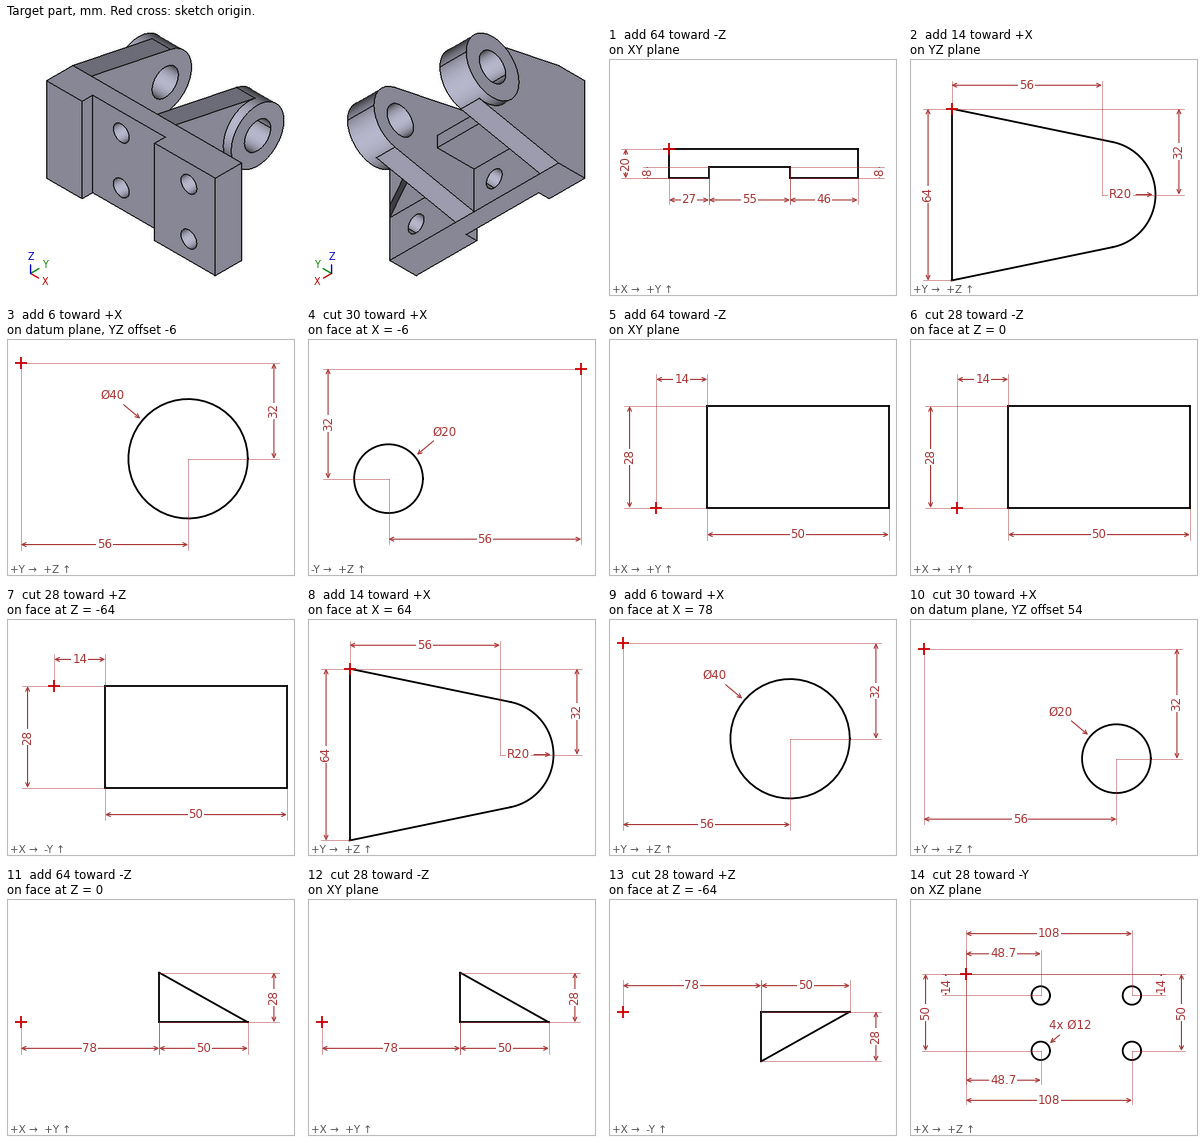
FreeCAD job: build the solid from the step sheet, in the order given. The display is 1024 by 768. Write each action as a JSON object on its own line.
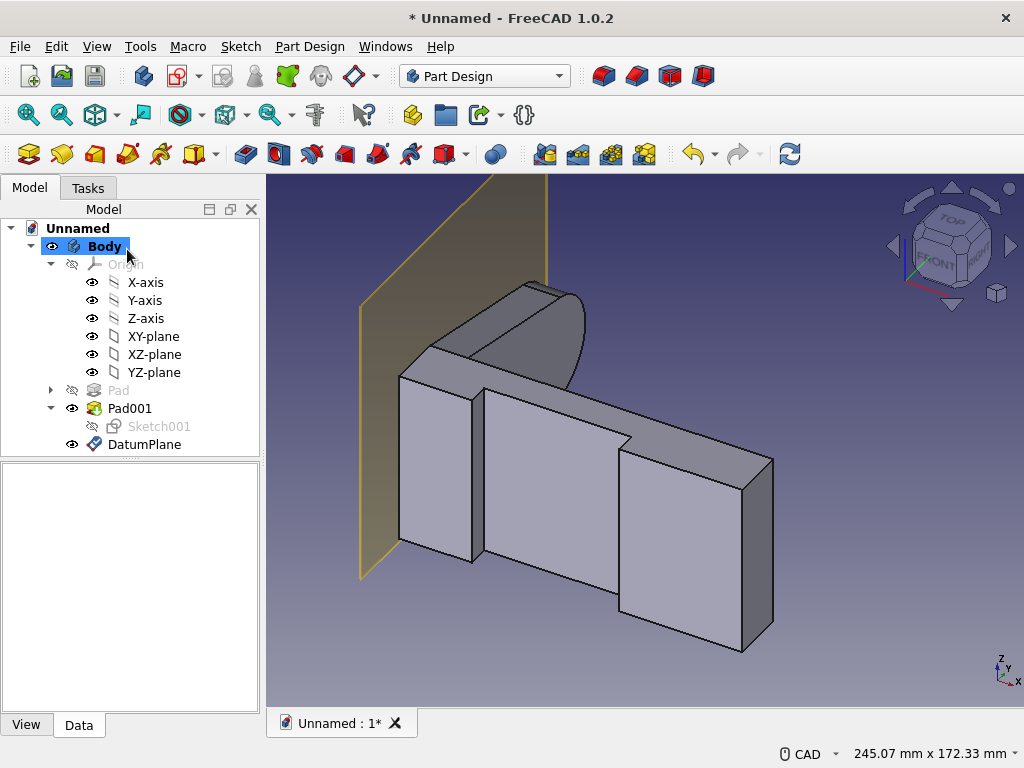
{"action": "left_click", "coordinate": [117, 444]}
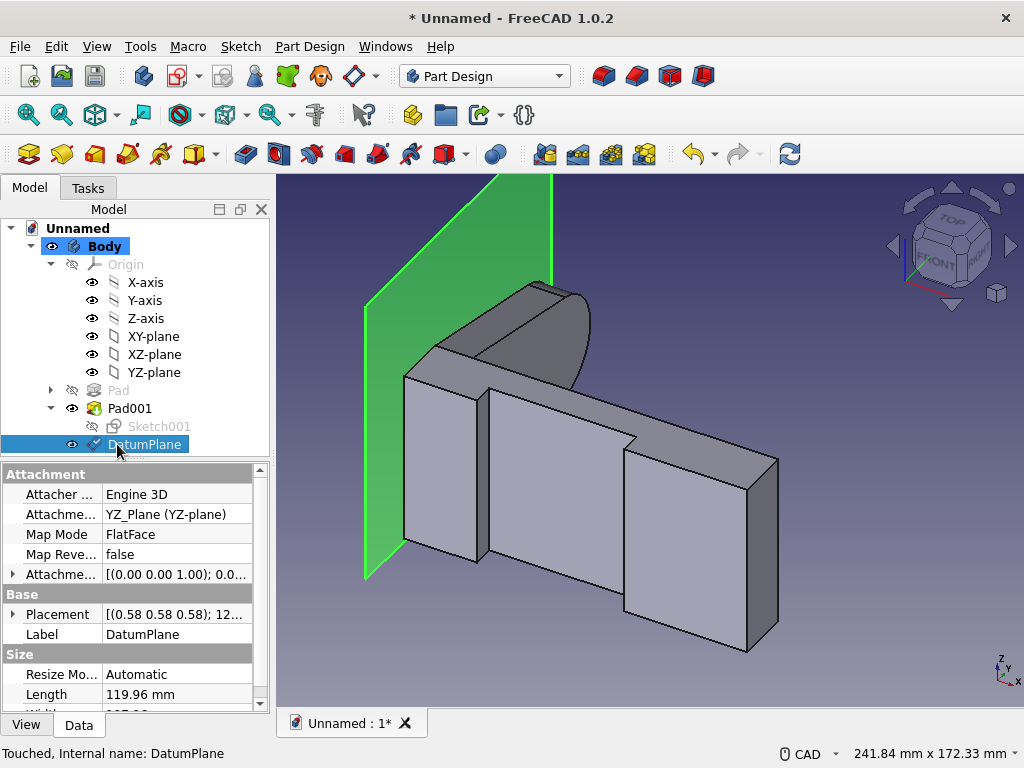
{"action": "left_click", "coordinate": [176, 76]}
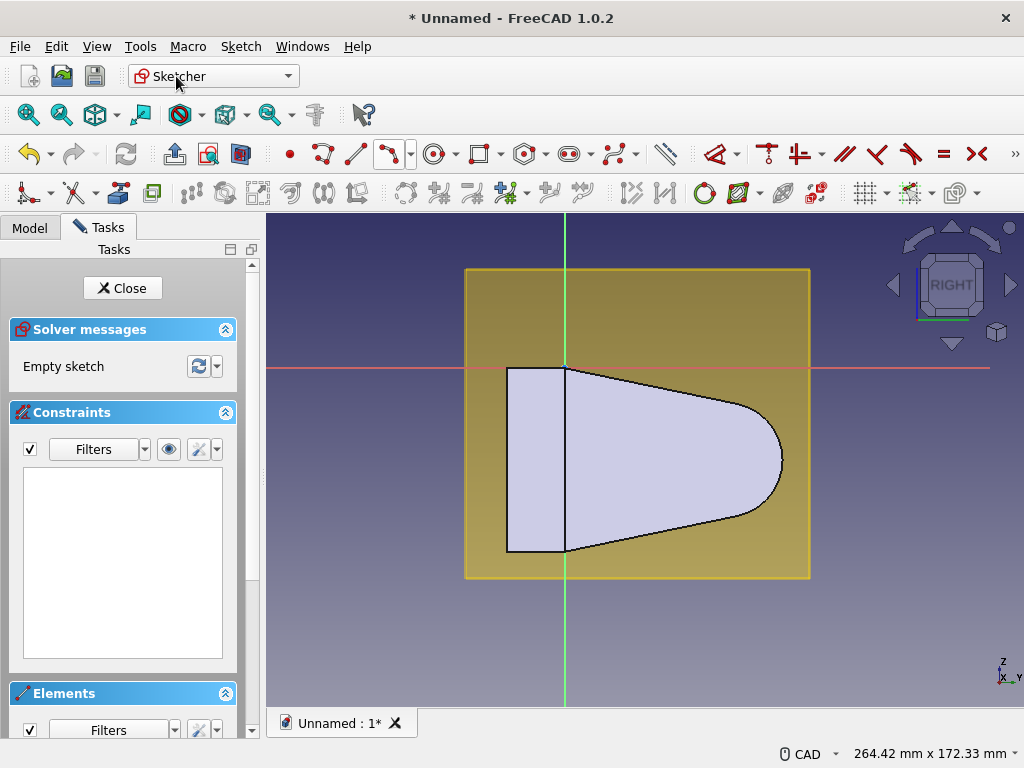
{"action": "left_click", "coordinate": [241, 154]}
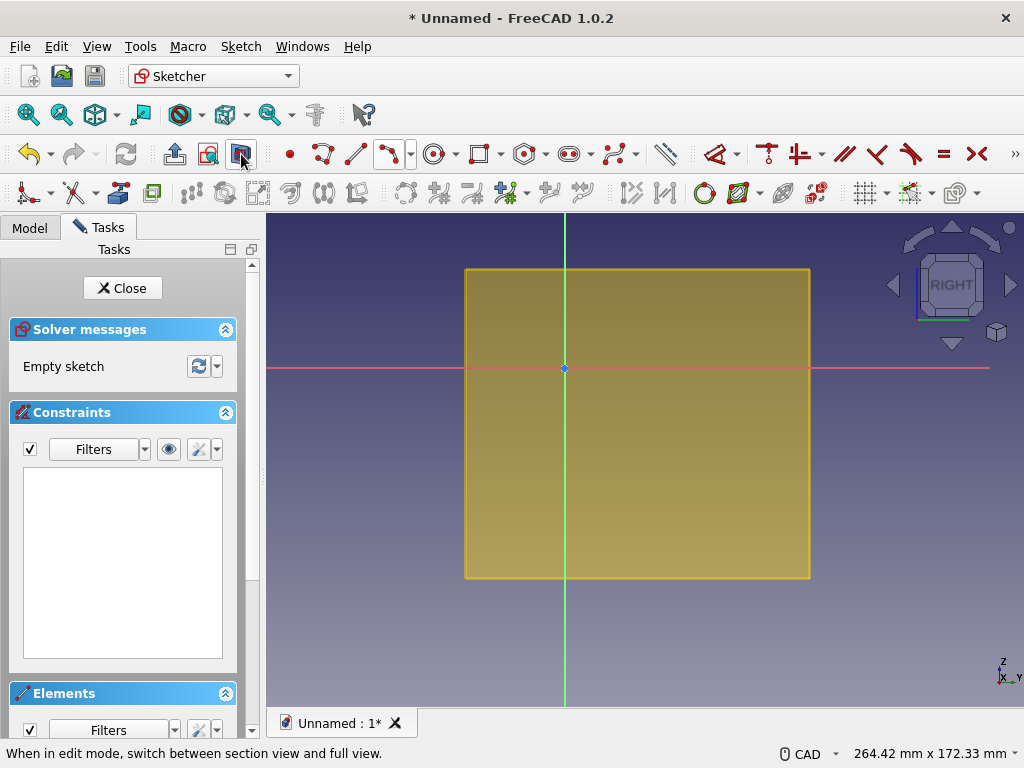
{"action": "scroll", "coordinate": [792, 422], "scroll_direction": "up", "scroll_amount": 3}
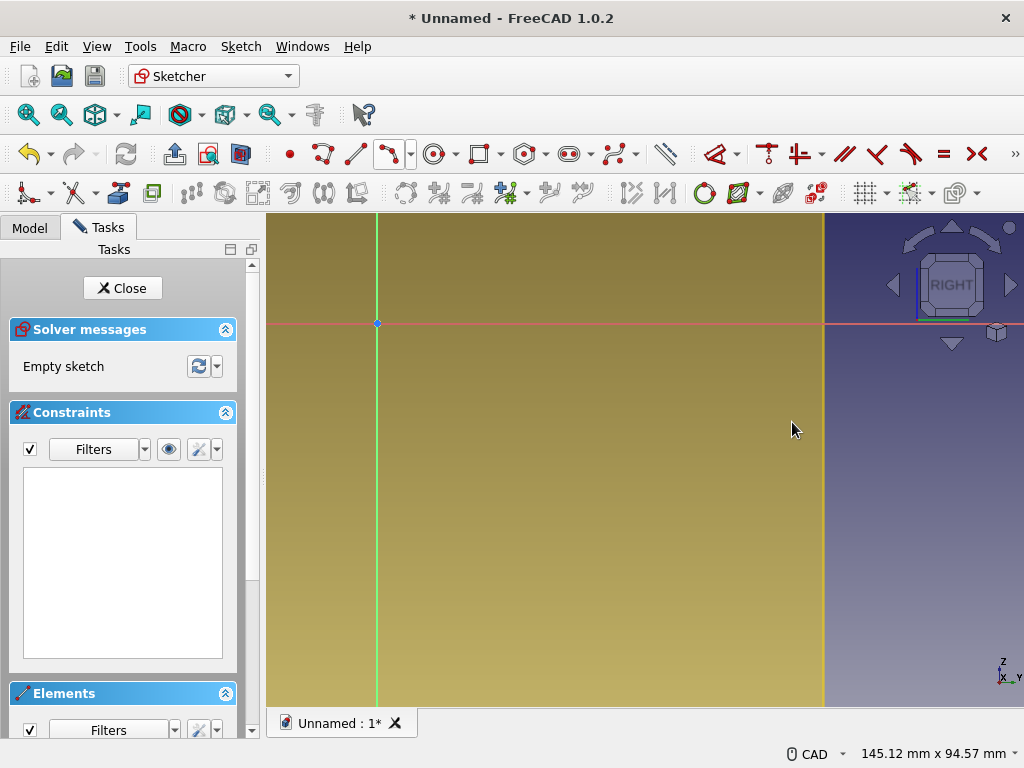
{"action": "left_click", "coordinate": [434, 154]}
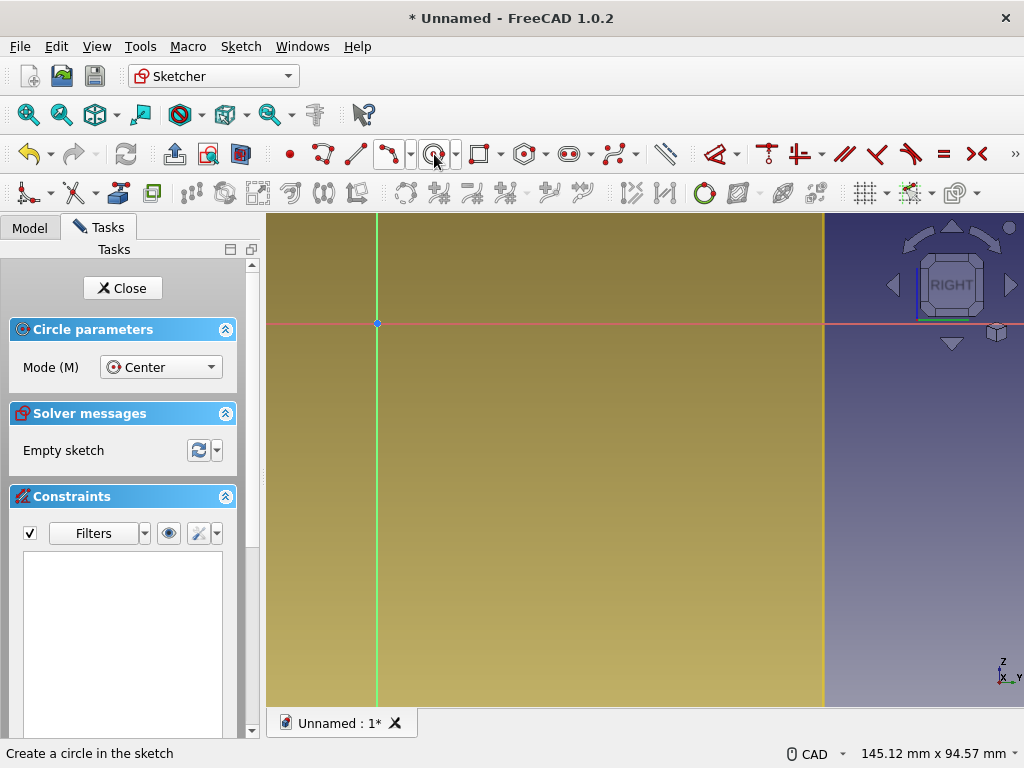
{"action": "left_click", "coordinate": [670, 491]}
{"action": "left_click", "coordinate": [744, 417]}
{"action": "key", "text": "Escape"}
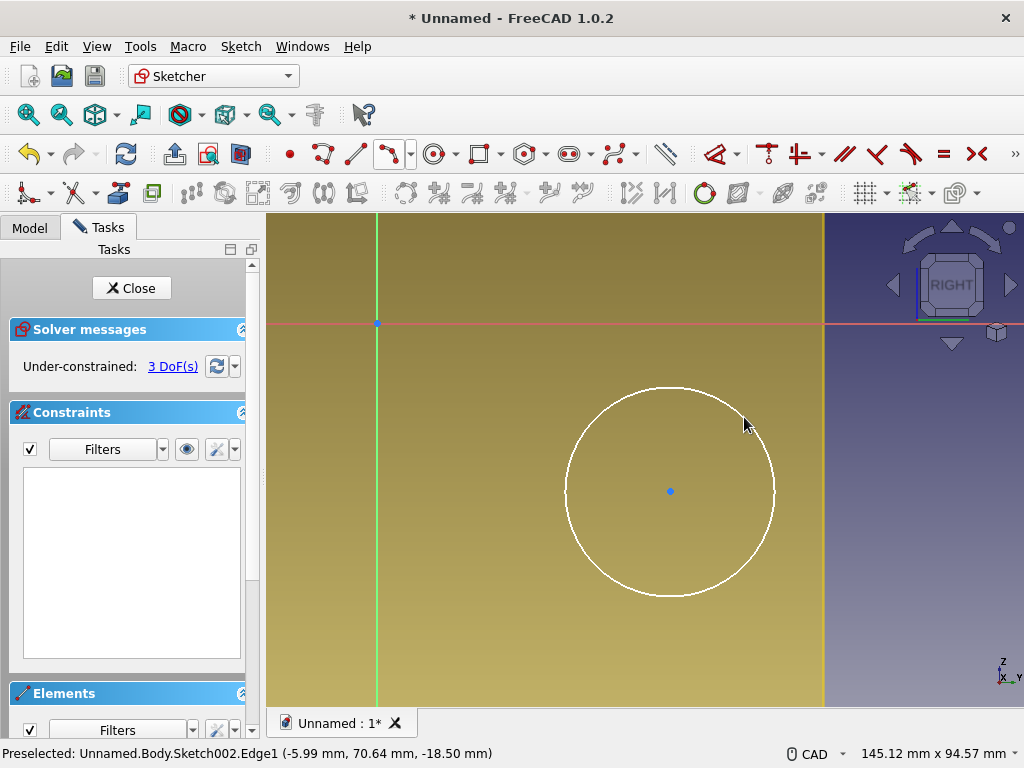
{"action": "left_click", "coordinate": [714, 154]}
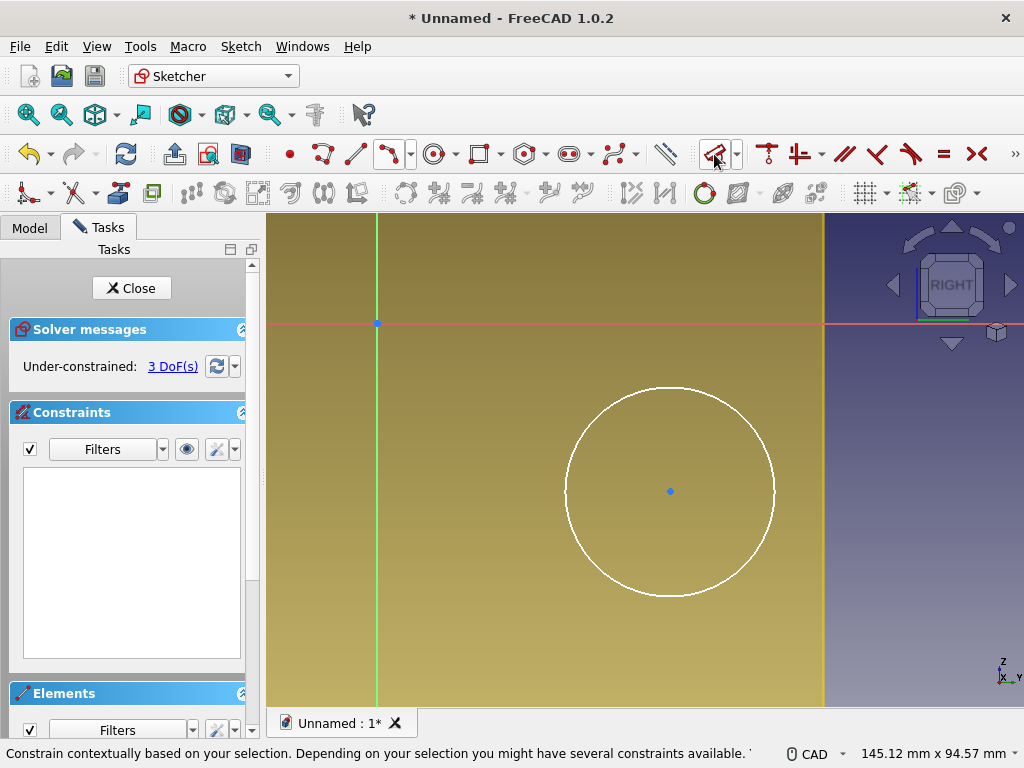
{"action": "left_click", "coordinate": [744, 418]}
{"action": "left_click", "coordinate": [767, 395]}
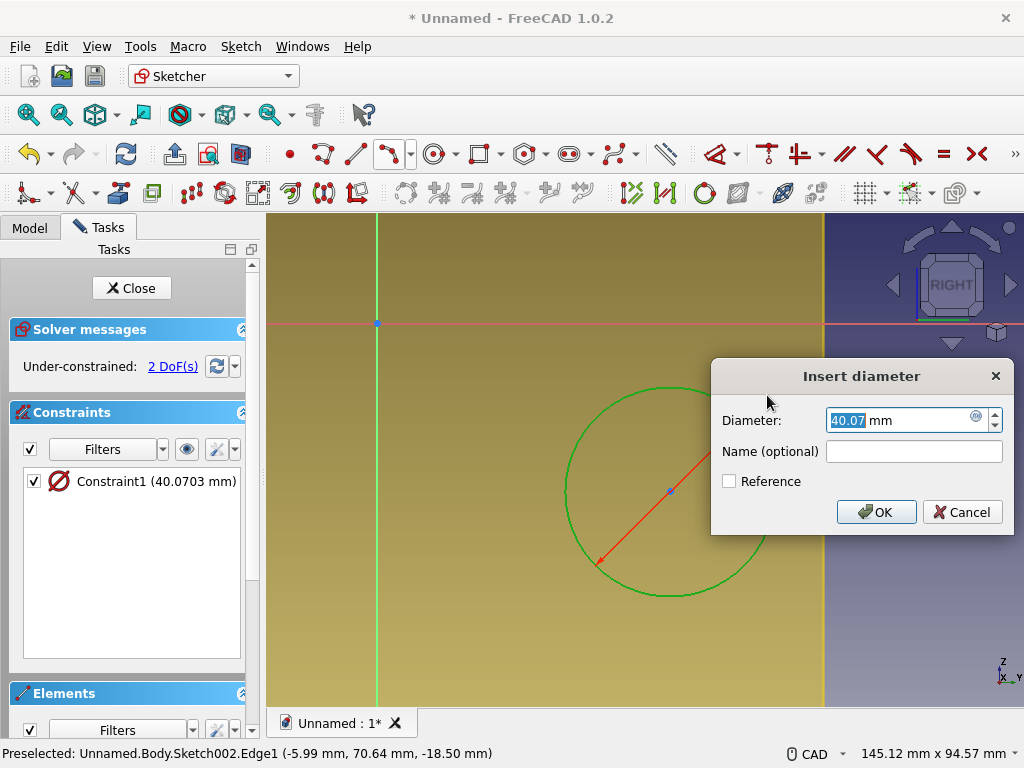
{"action": "type", "text": "40"}
{"action": "key", "text": "Return"}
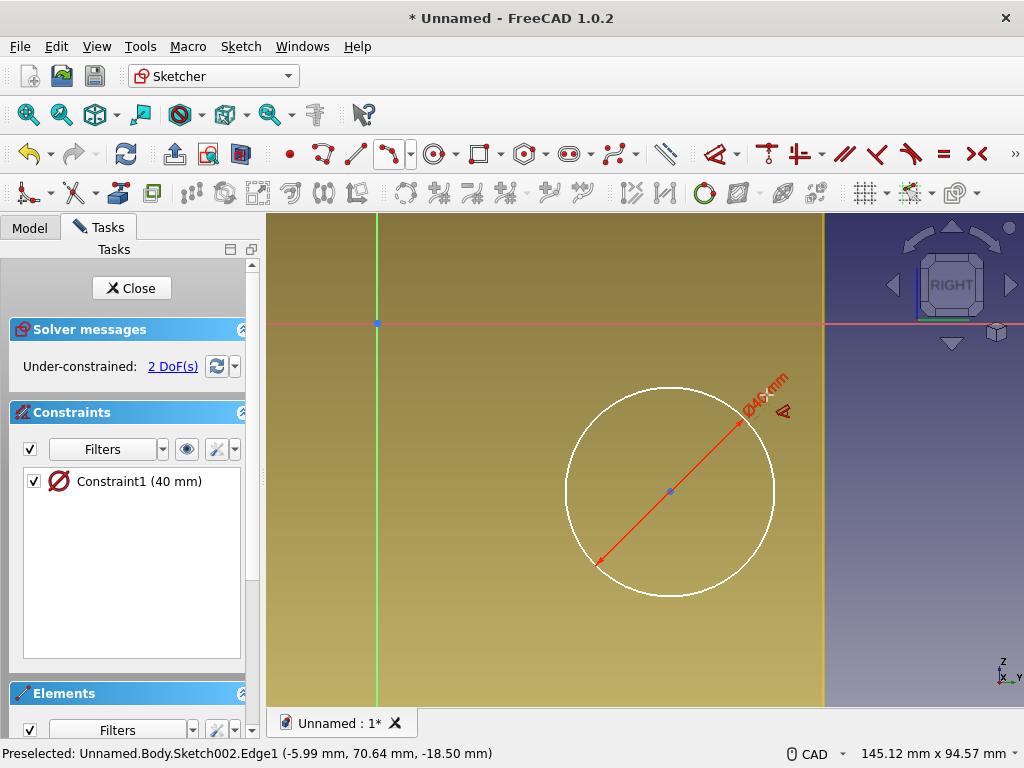
{"action": "left_click", "coordinate": [670, 492]}
{"action": "left_click", "coordinate": [524, 290]}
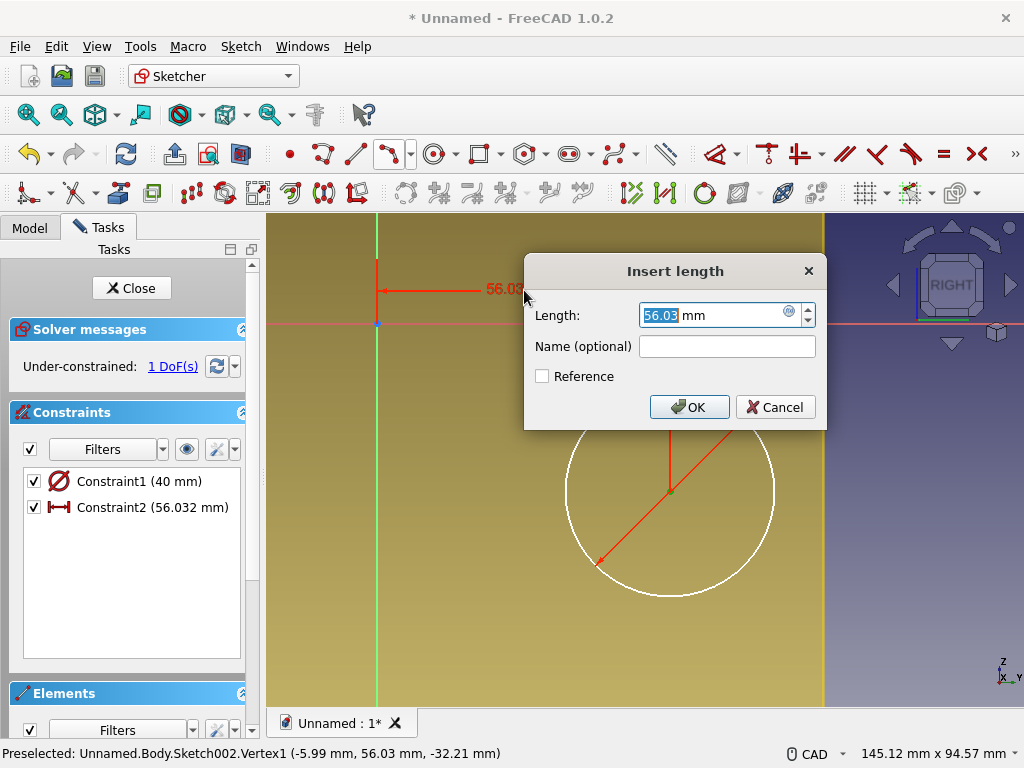
{"action": "type", "text": "56"}
{"action": "key", "text": "Return"}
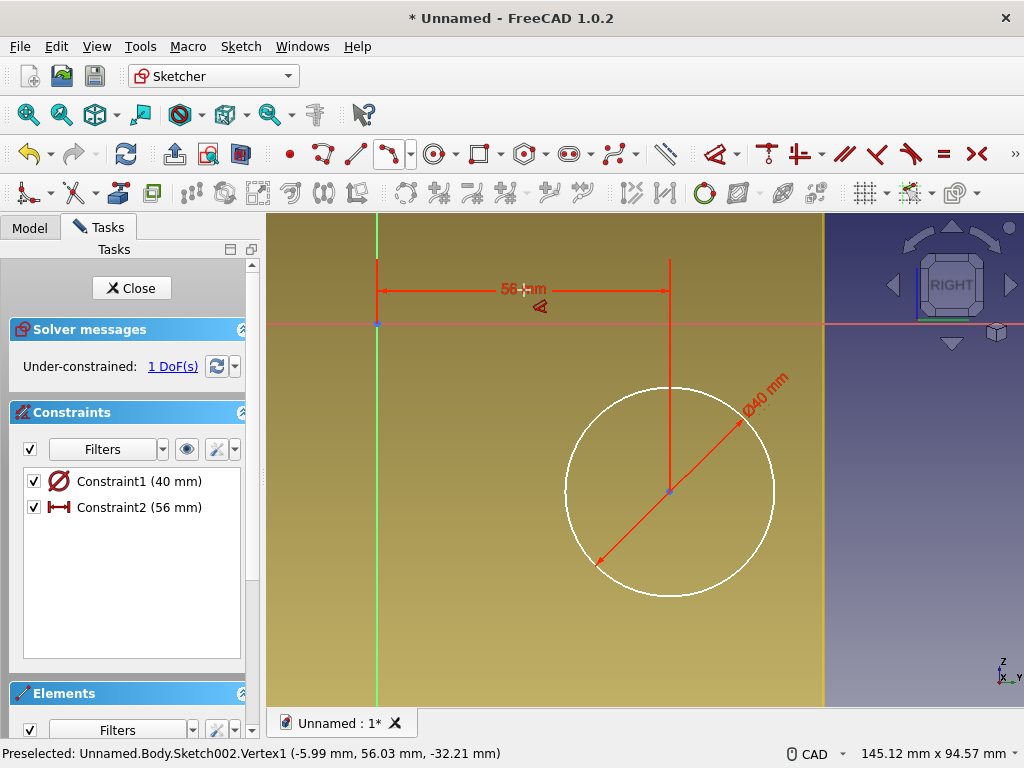
{"action": "left_click", "coordinate": [670, 492]}
{"action": "left_click", "coordinate": [343, 408]}